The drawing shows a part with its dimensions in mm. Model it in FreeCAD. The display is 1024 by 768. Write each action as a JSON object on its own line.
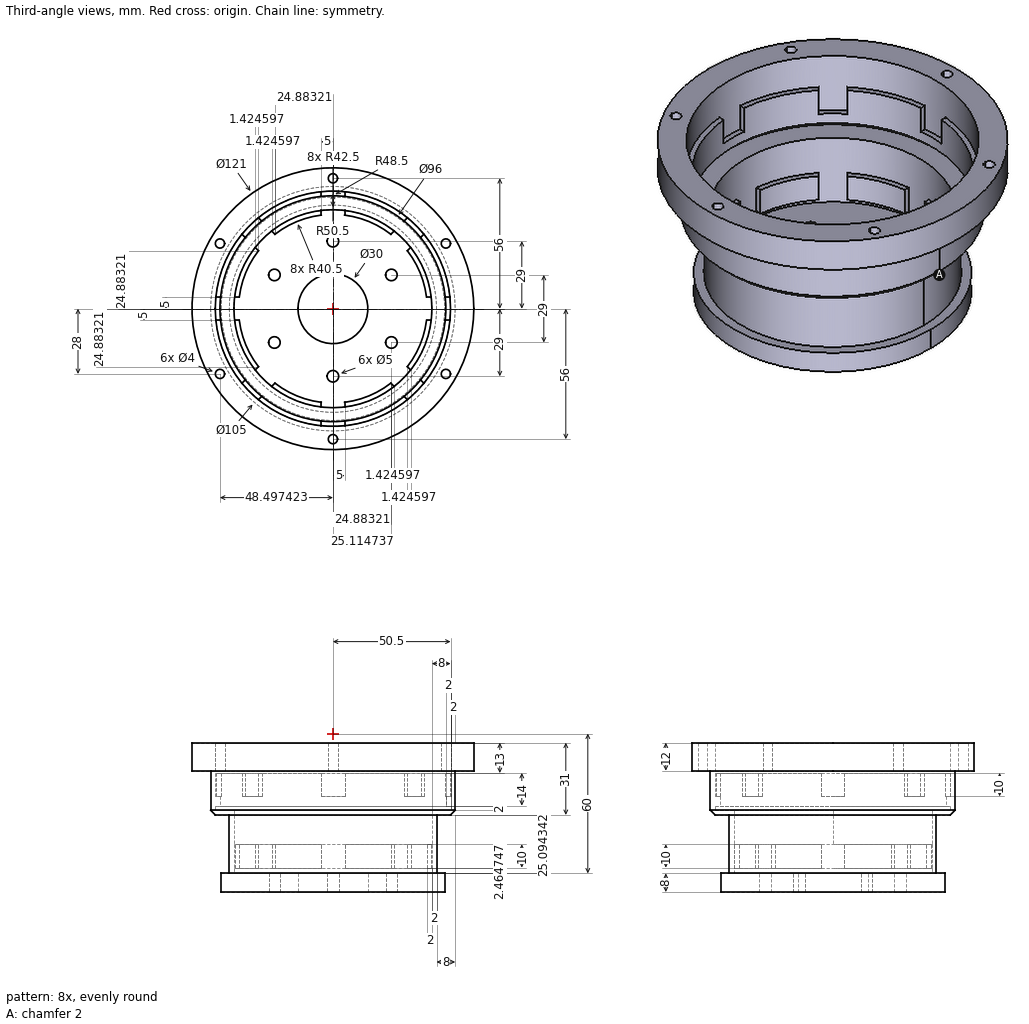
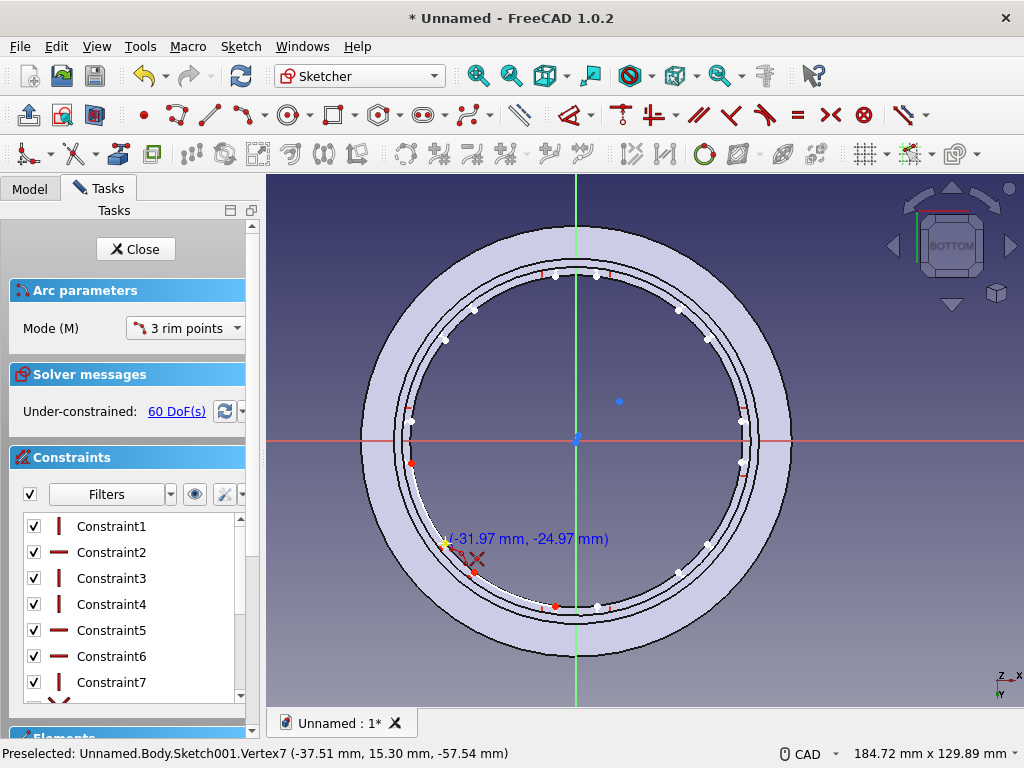
{"action": "scroll", "coordinate": [403, 462], "scroll_direction": "up", "scroll_amount": 7}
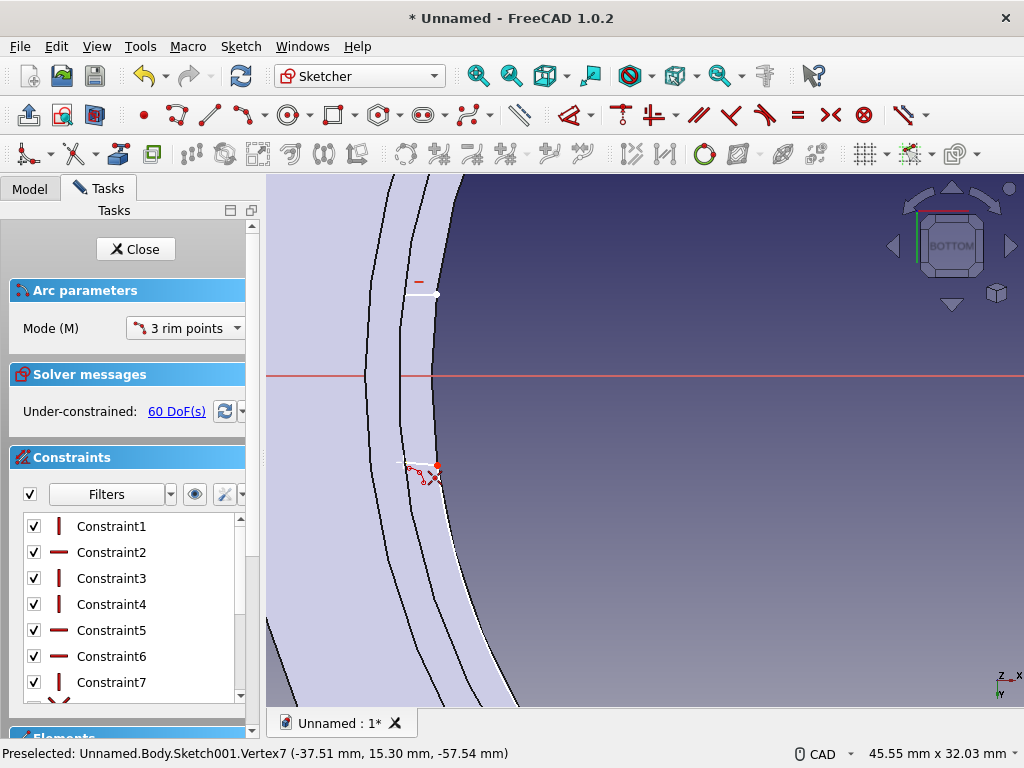
{"action": "left_click", "coordinate": [404, 462]}
{"action": "left_click", "coordinate": [404, 295]}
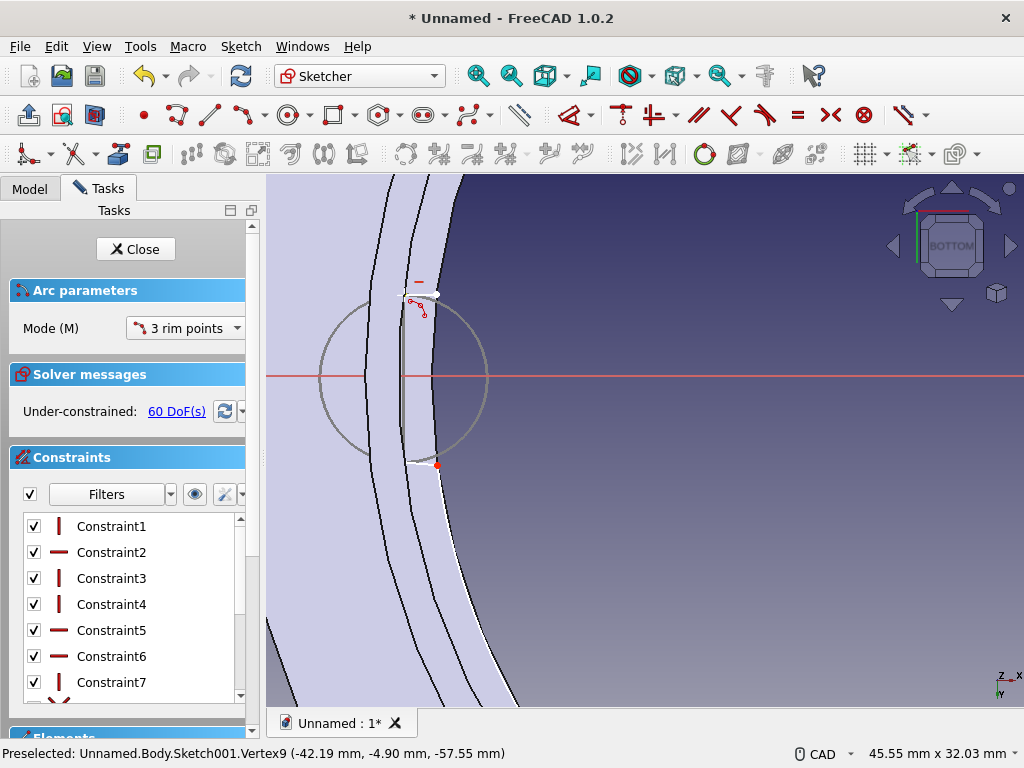
{"action": "scroll", "coordinate": [399, 360], "scroll_direction": "up", "scroll_amount": 7}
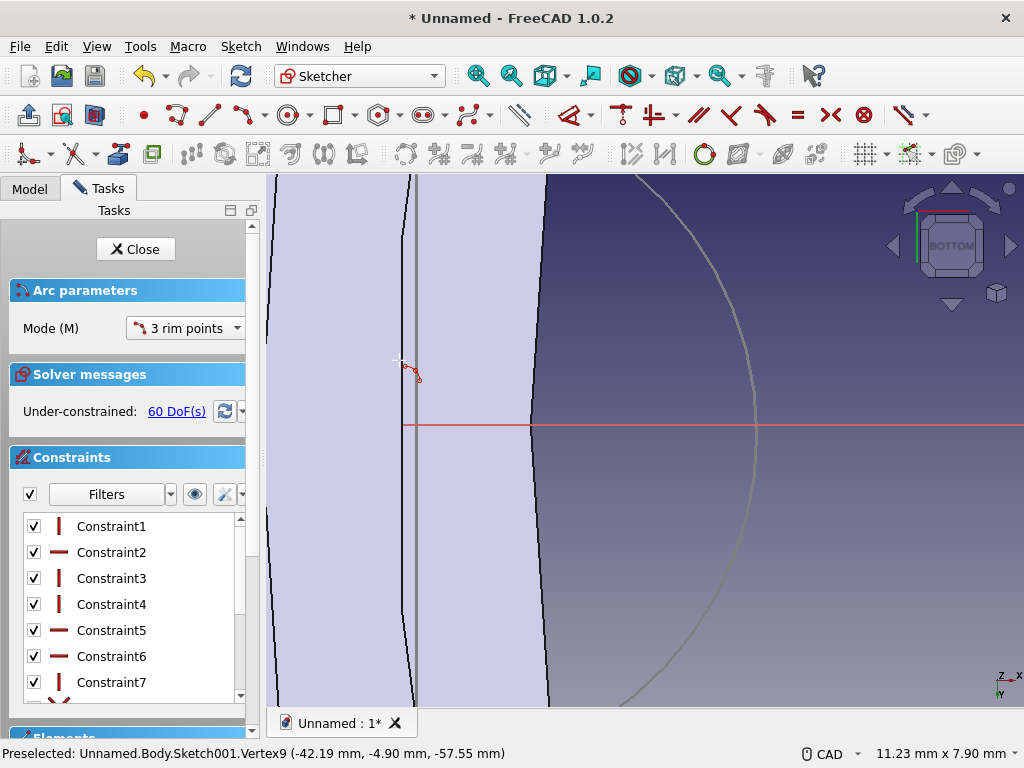
{"action": "left_click", "coordinate": [397, 358]}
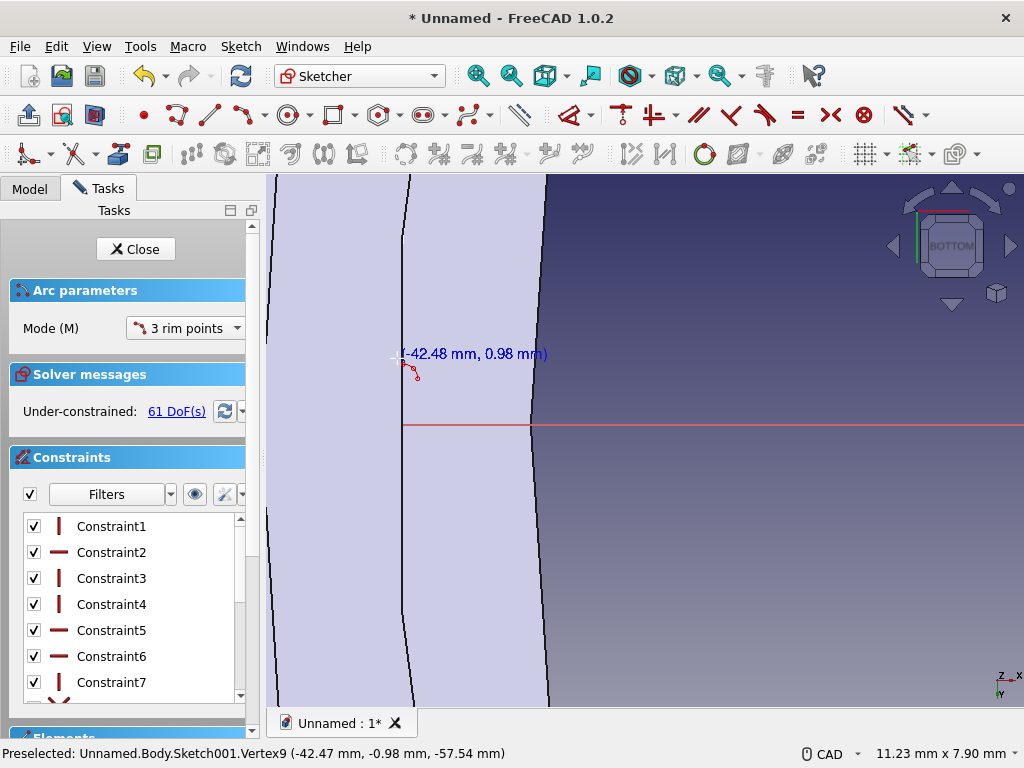
{"action": "scroll", "coordinate": [403, 441], "scroll_direction": "down", "scroll_amount": 14}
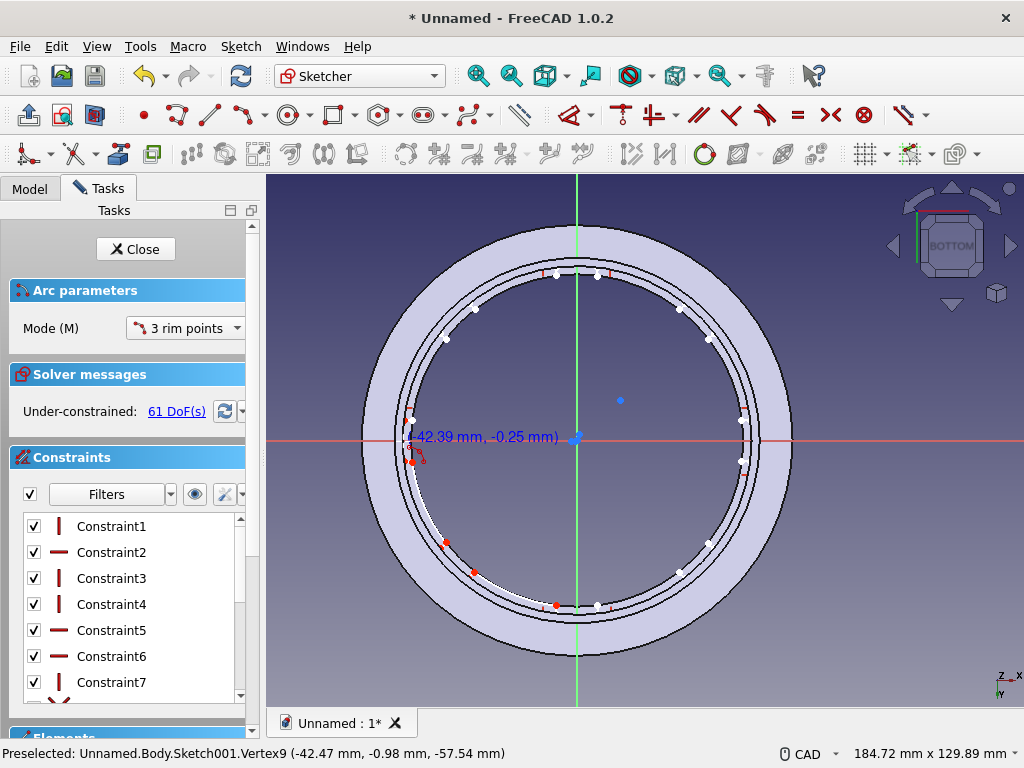
{"action": "scroll", "coordinate": [412, 420], "scroll_direction": "up", "scroll_amount": 7}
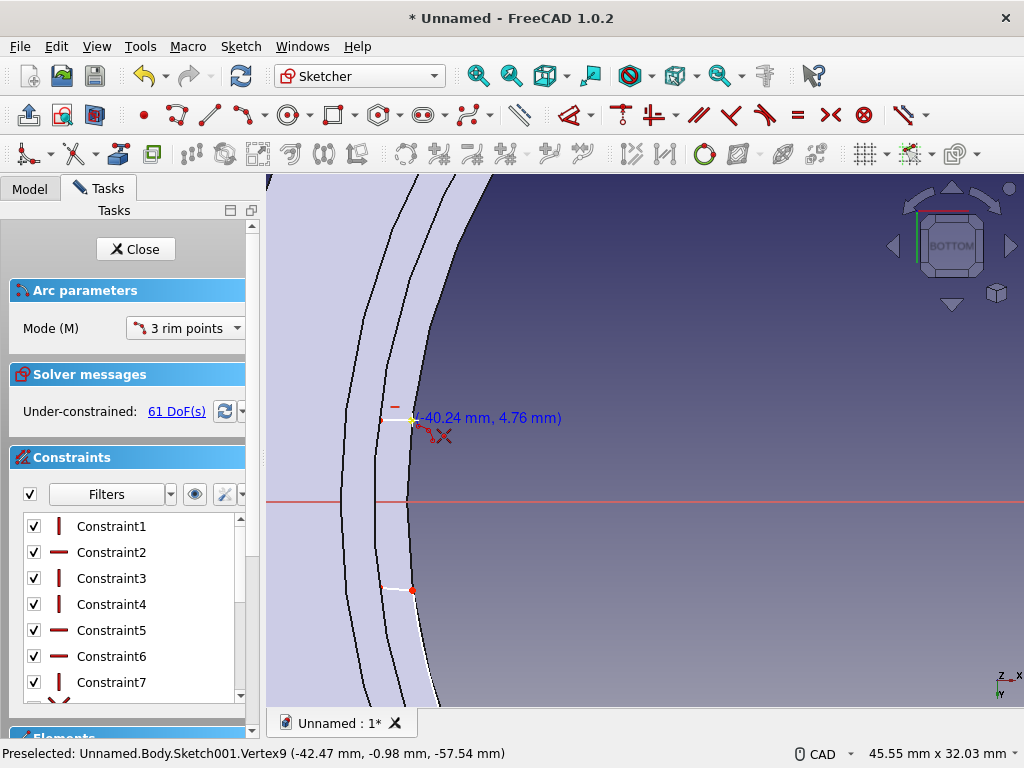
{"action": "left_click", "coordinate": [412, 420]}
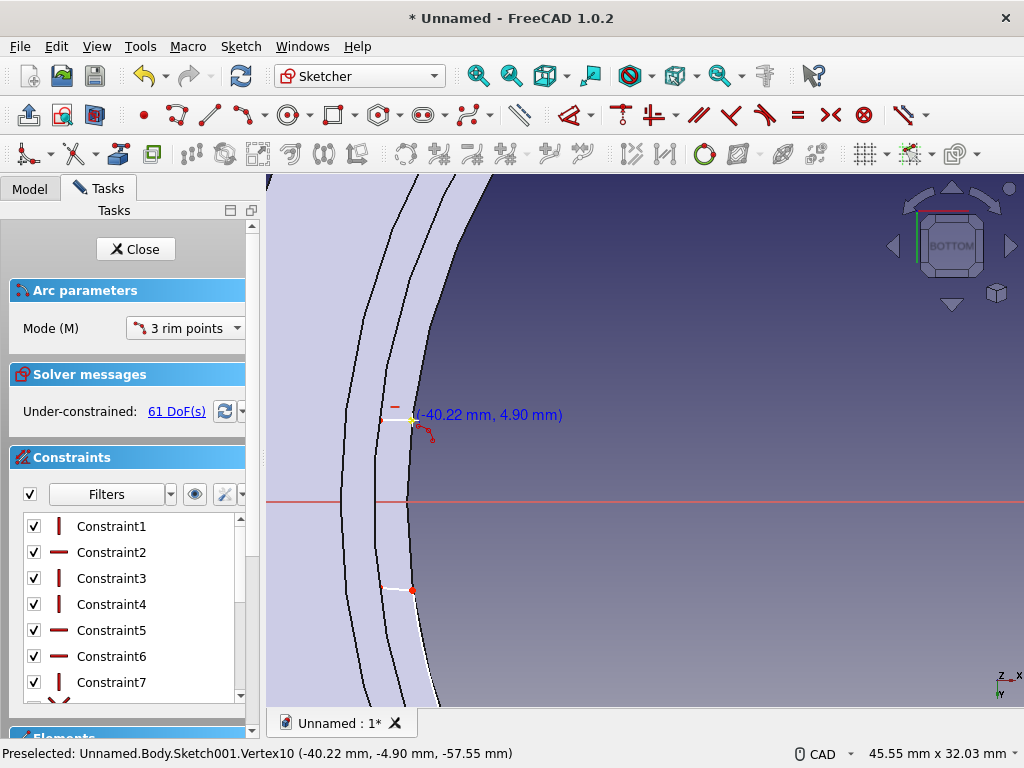
{"action": "scroll", "coordinate": [411, 420], "scroll_direction": "down", "scroll_amount": 7}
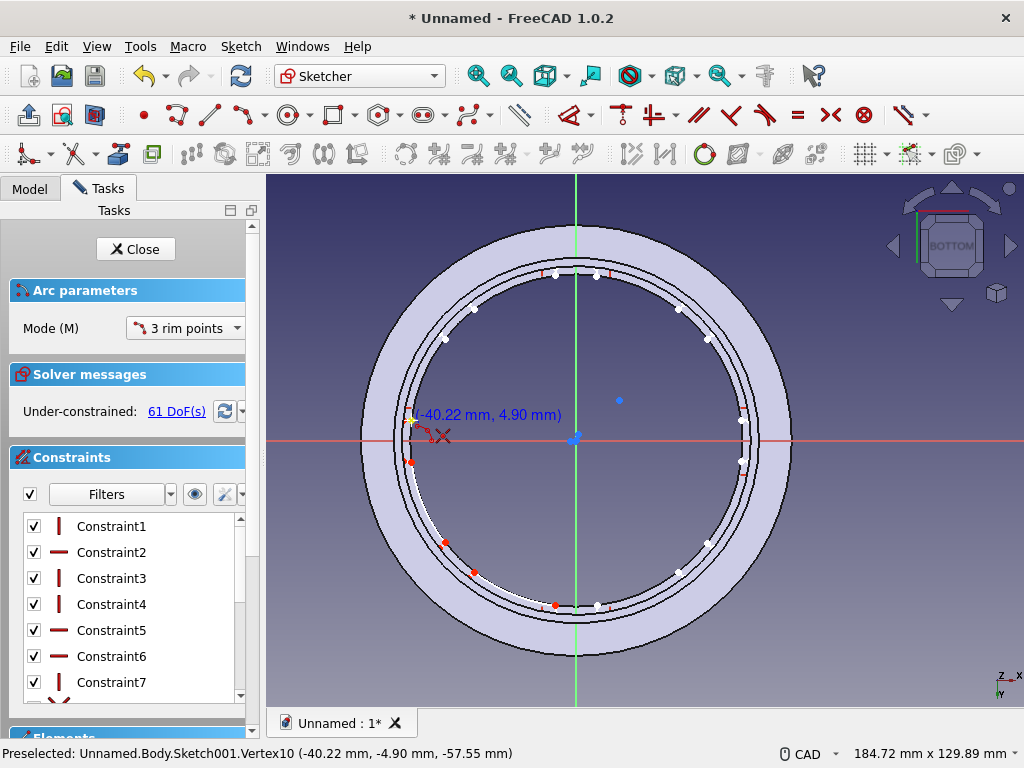
{"action": "scroll", "coordinate": [445, 338], "scroll_direction": "up", "scroll_amount": 7}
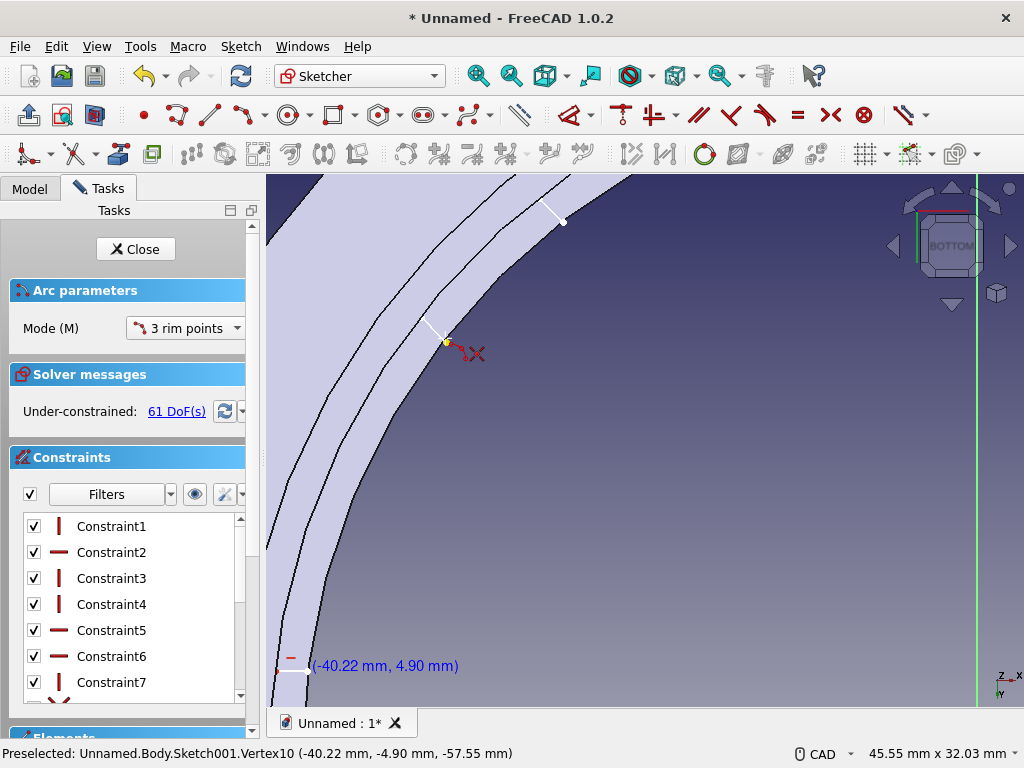
{"action": "left_click", "coordinate": [447, 343]}
{"action": "left_click", "coordinate": [354, 495]}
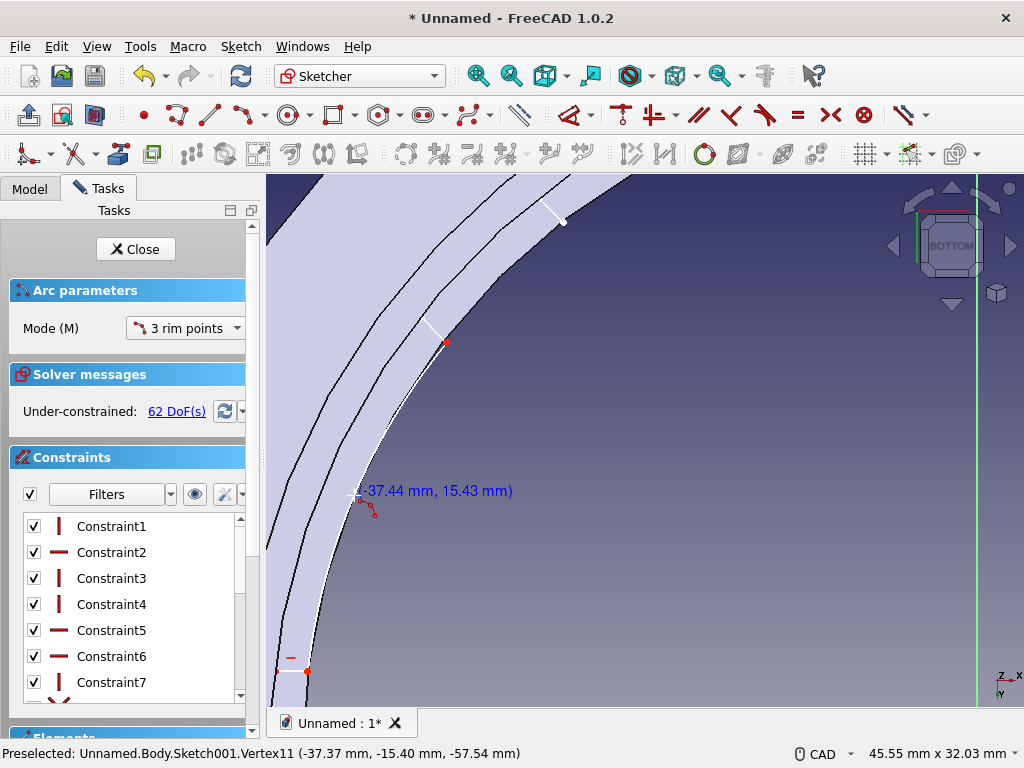
{"action": "left_click", "coordinate": [421, 317]}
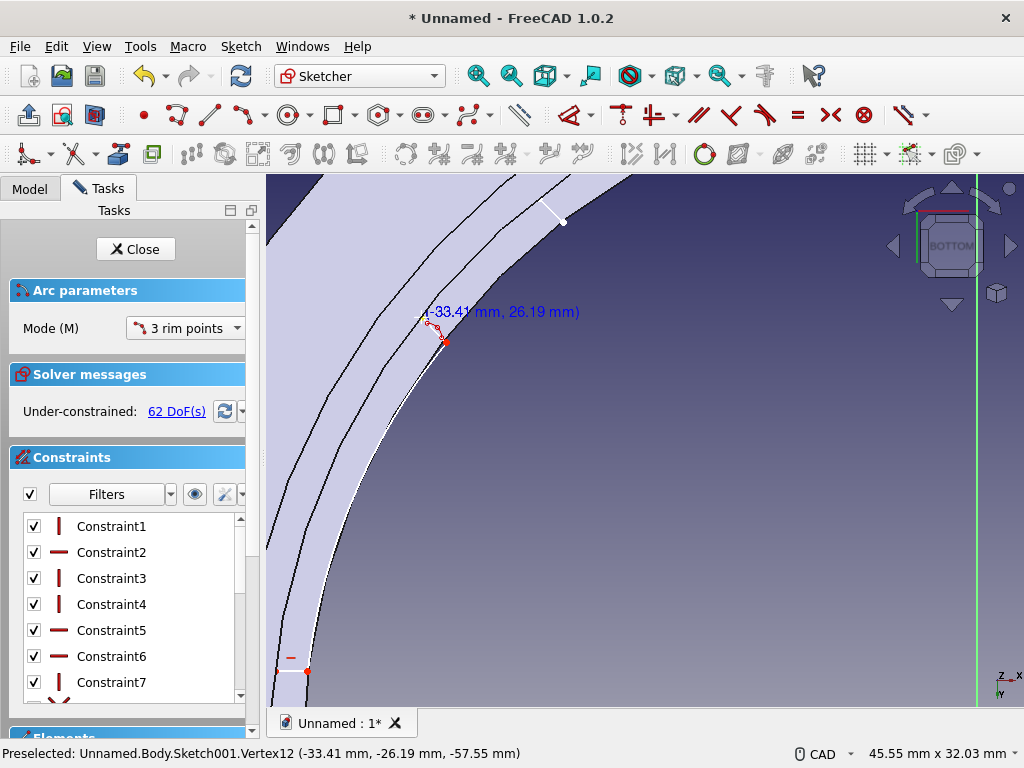
{"action": "scroll", "coordinate": [445, 338], "scroll_direction": "down", "scroll_amount": 7}